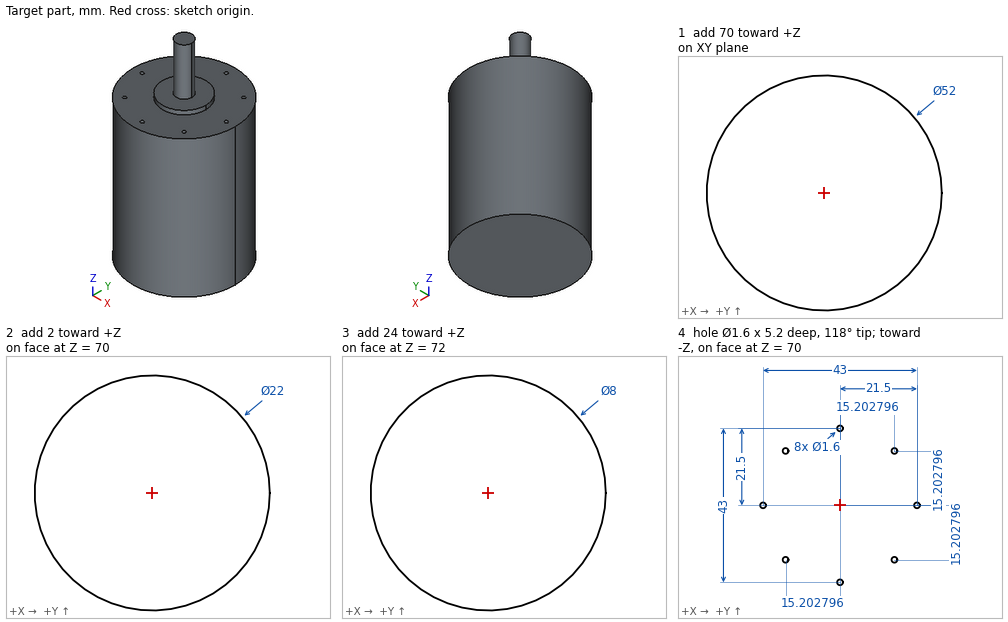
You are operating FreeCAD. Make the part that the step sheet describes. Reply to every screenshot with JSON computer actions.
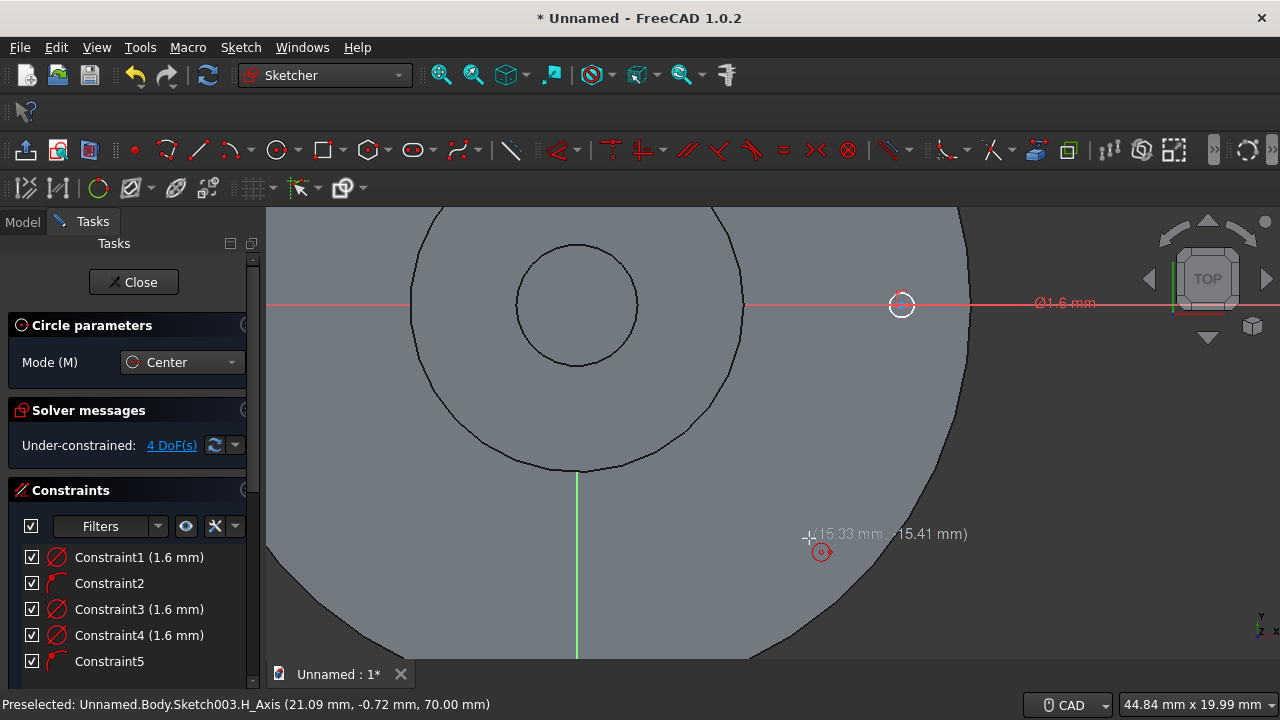
{"action": "left_click", "coordinate": [809, 537]}
{"action": "mouse_move", "coordinate": [812, 534]}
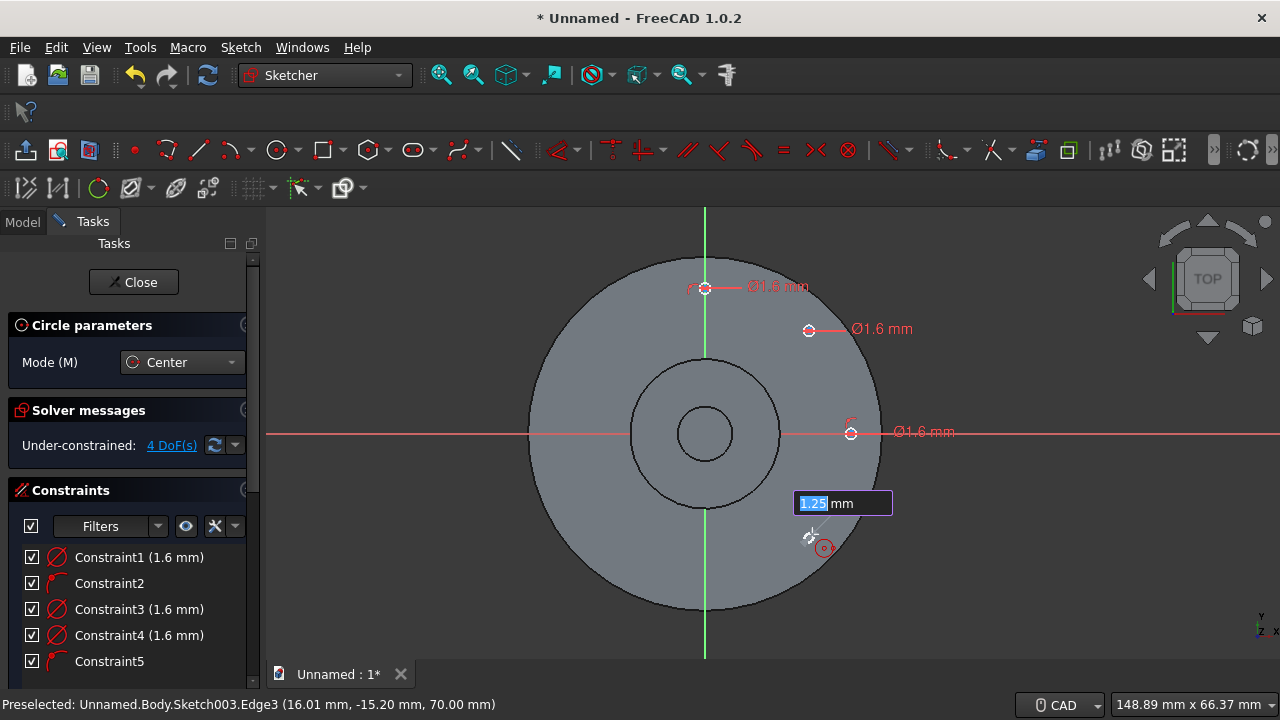
{"action": "type", "text": "1.6"}
{"action": "key", "text": "Return"}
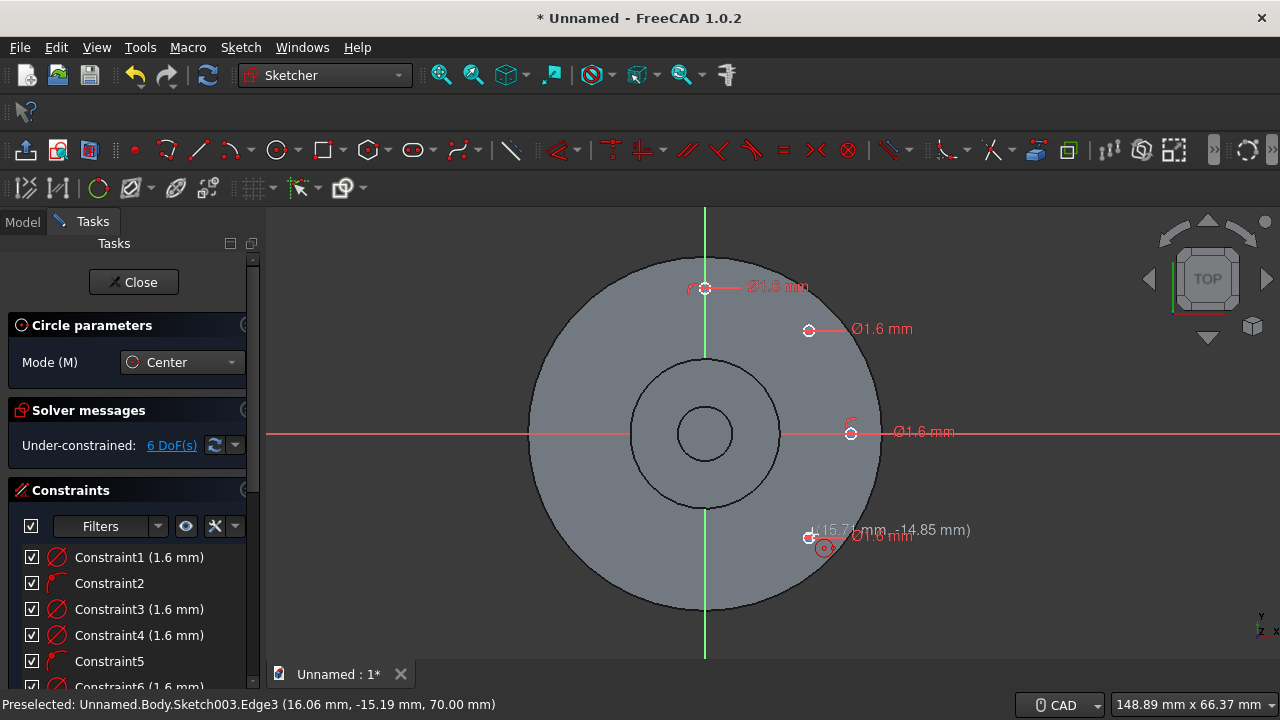
{"action": "scroll", "coordinate": [705, 580], "scroll_direction": "up", "scroll_amount": 8}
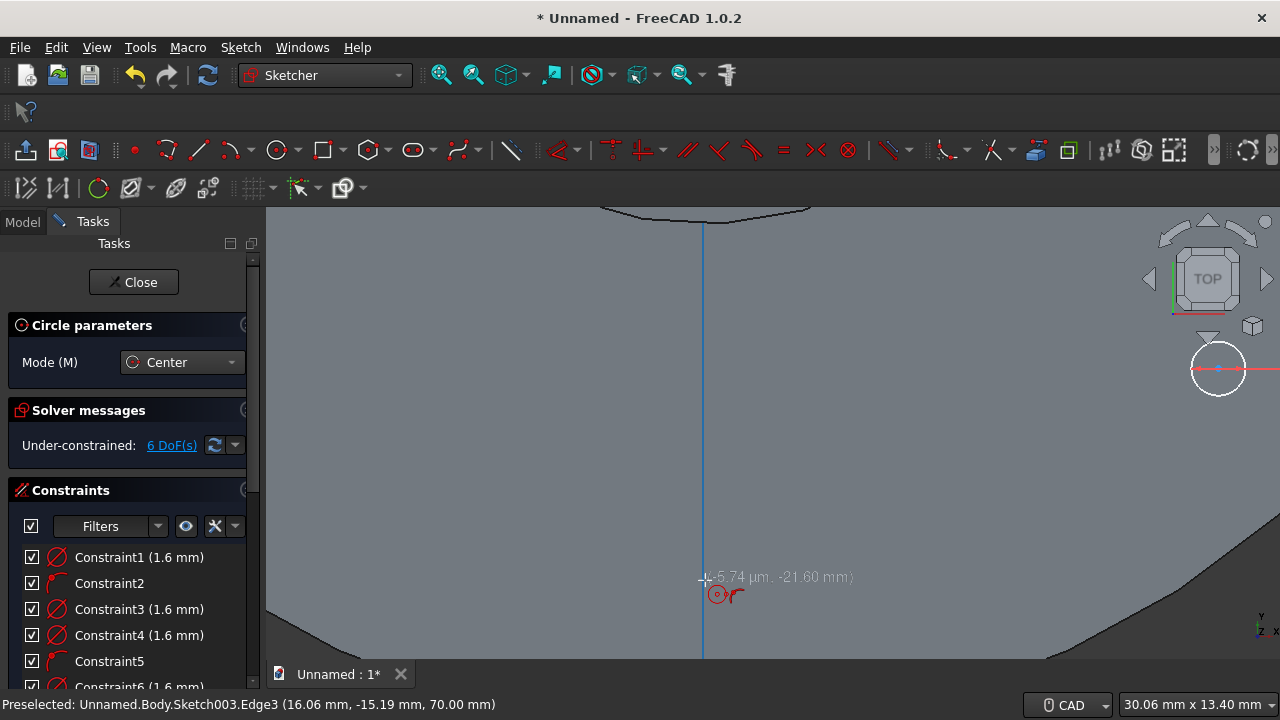
{"action": "scroll", "coordinate": [705, 580], "scroll_direction": "down", "scroll_amount": 8}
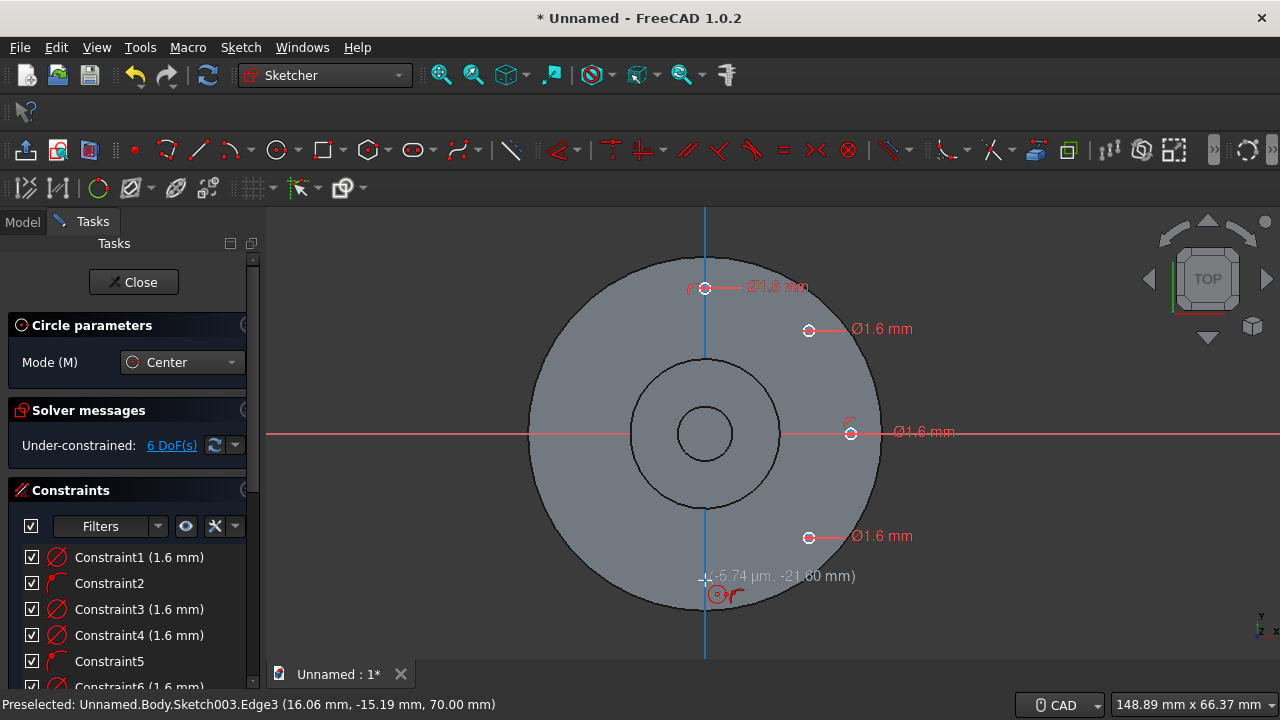
{"action": "left_click", "coordinate": [705, 580]}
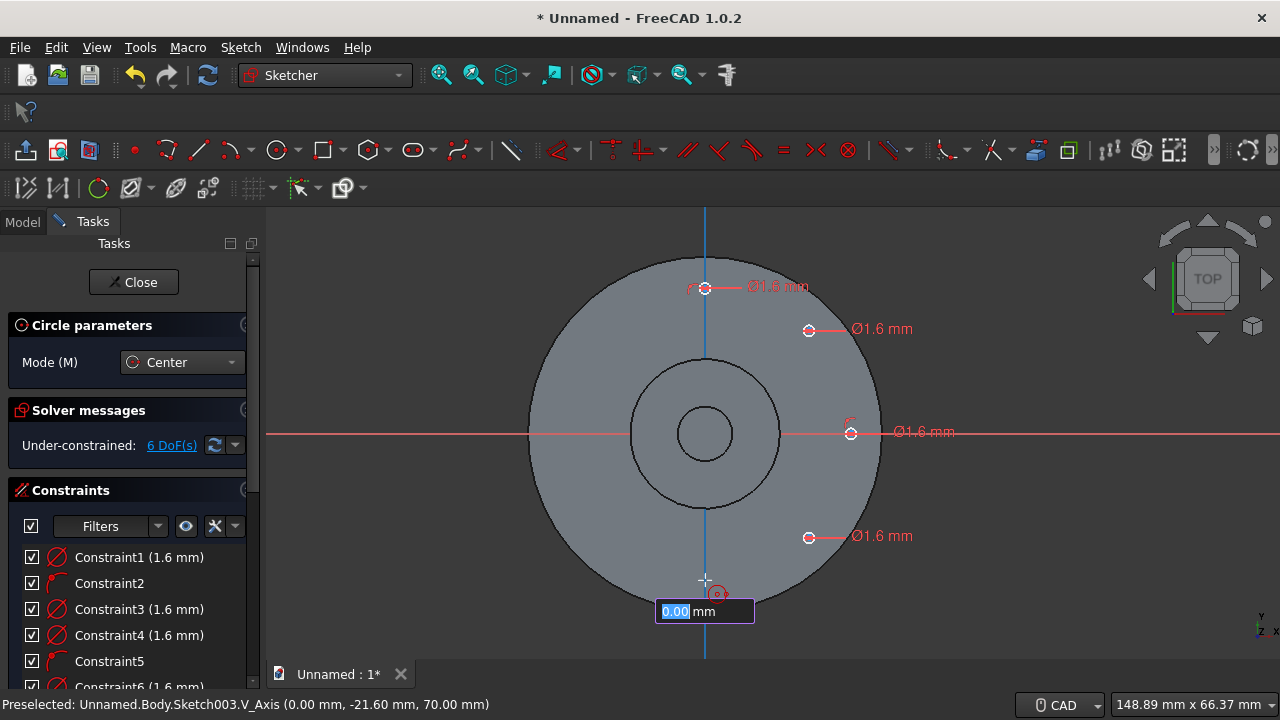
{"action": "scroll", "coordinate": [710, 578], "scroll_direction": "up", "scroll_amount": 6}
{"action": "mouse_move", "coordinate": [710, 577]}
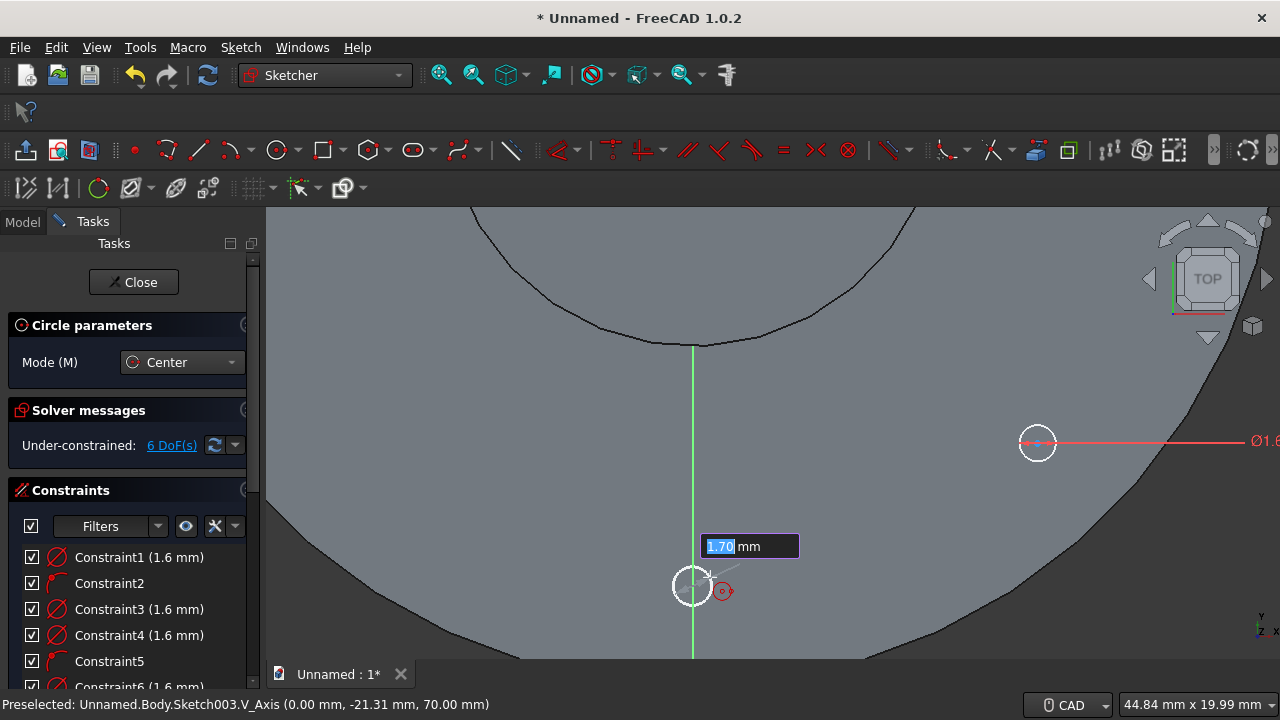
{"action": "type", "text": "1.6"}
{"action": "key", "text": "Return"}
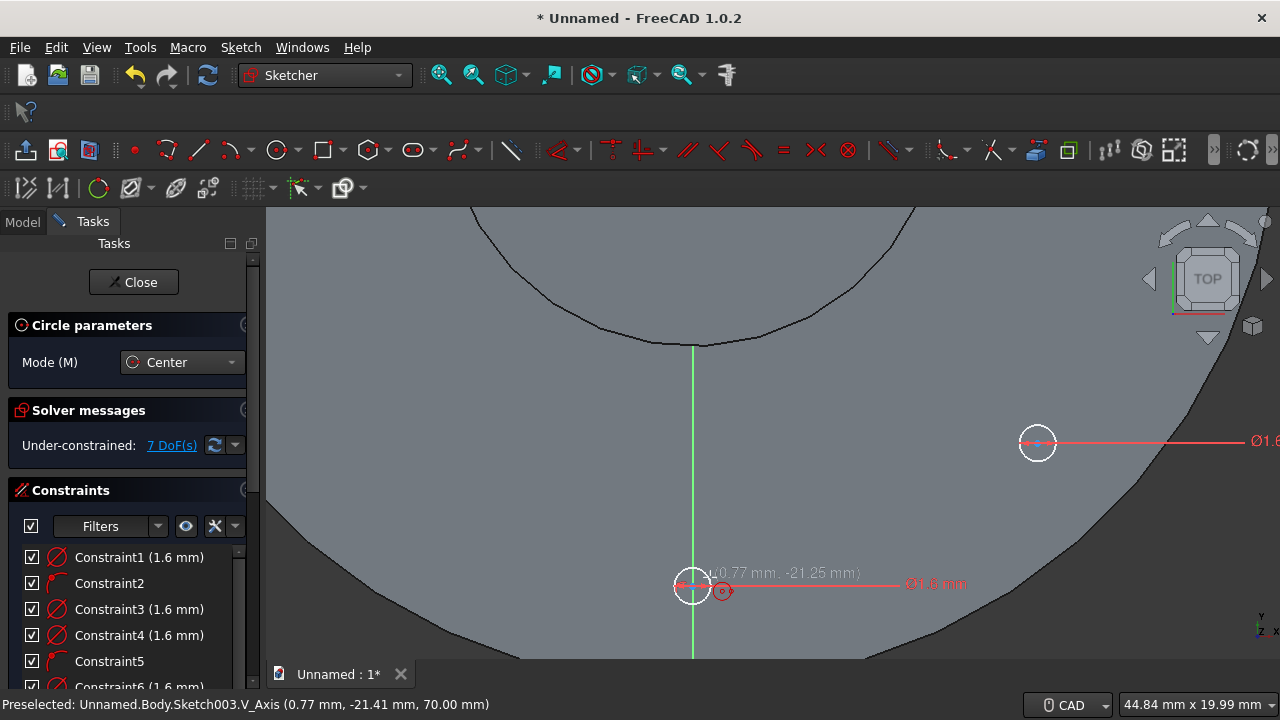
{"action": "scroll", "coordinate": [349, 441], "scroll_direction": "up", "scroll_amount": 2}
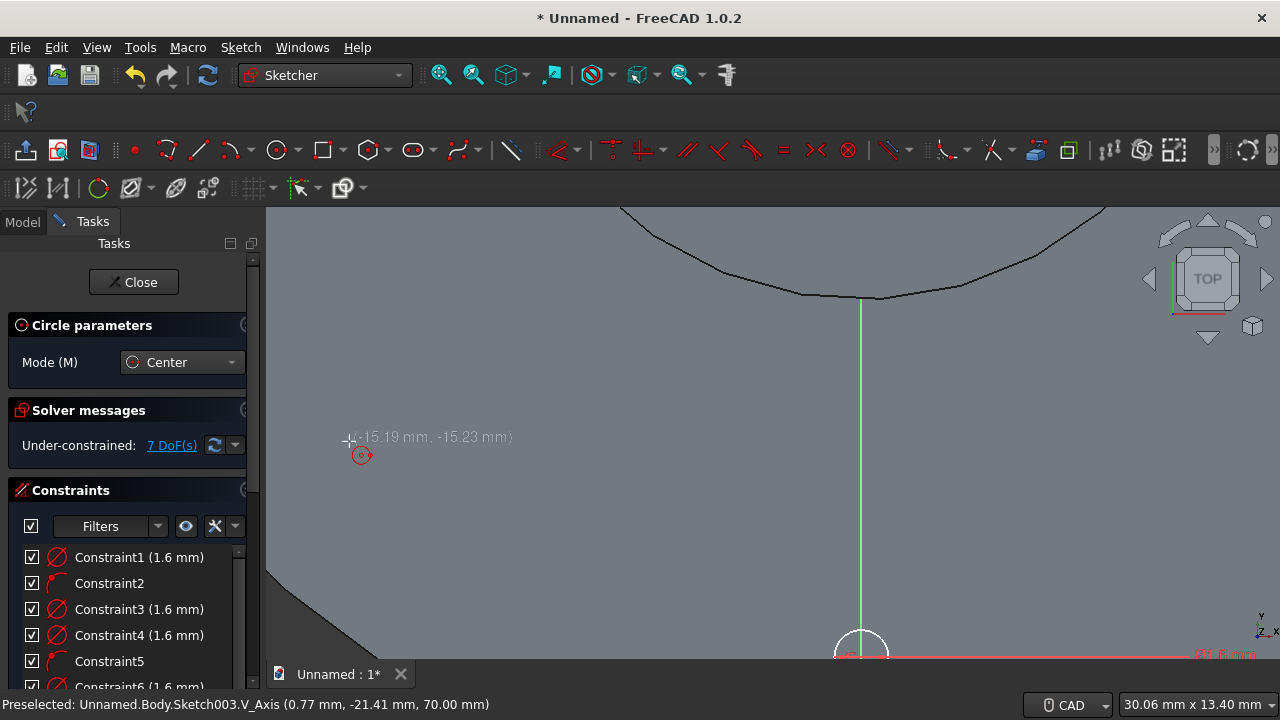
{"action": "scroll", "coordinate": [665, 561], "scroll_direction": "down", "scroll_amount": 8}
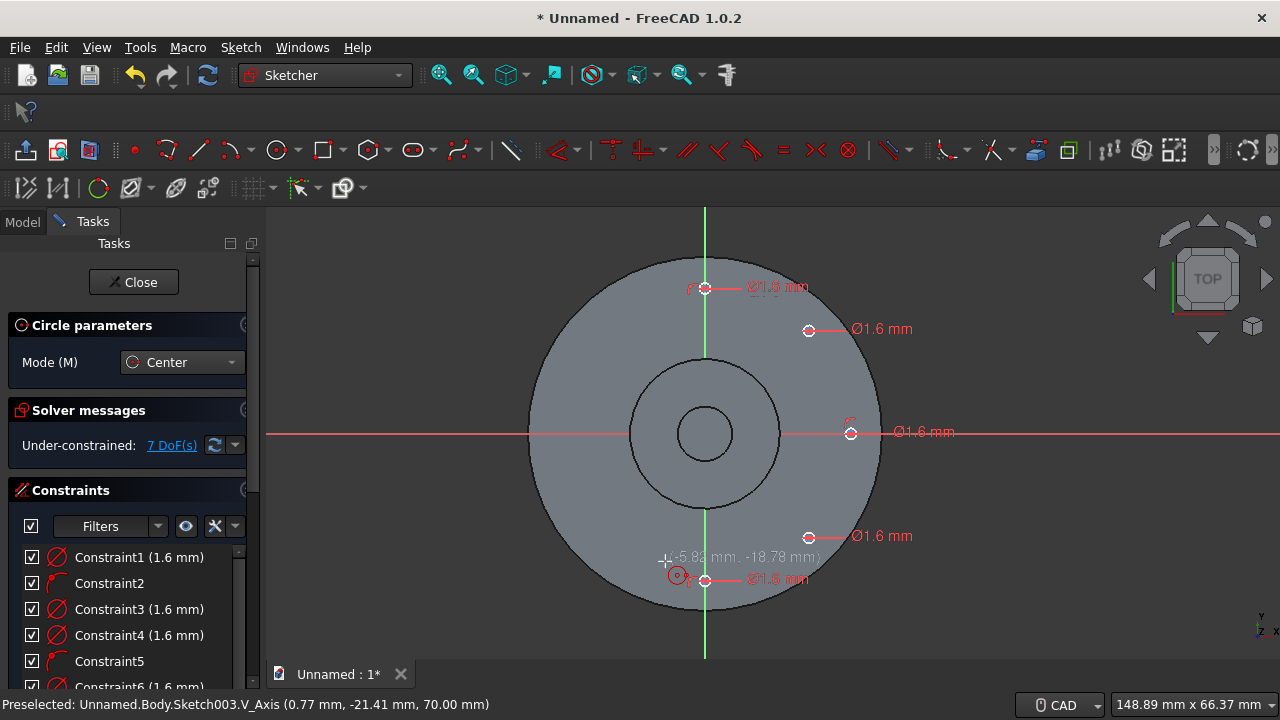
{"action": "left_click", "coordinate": [601, 537]}
{"action": "mouse_move", "coordinate": [605, 534]}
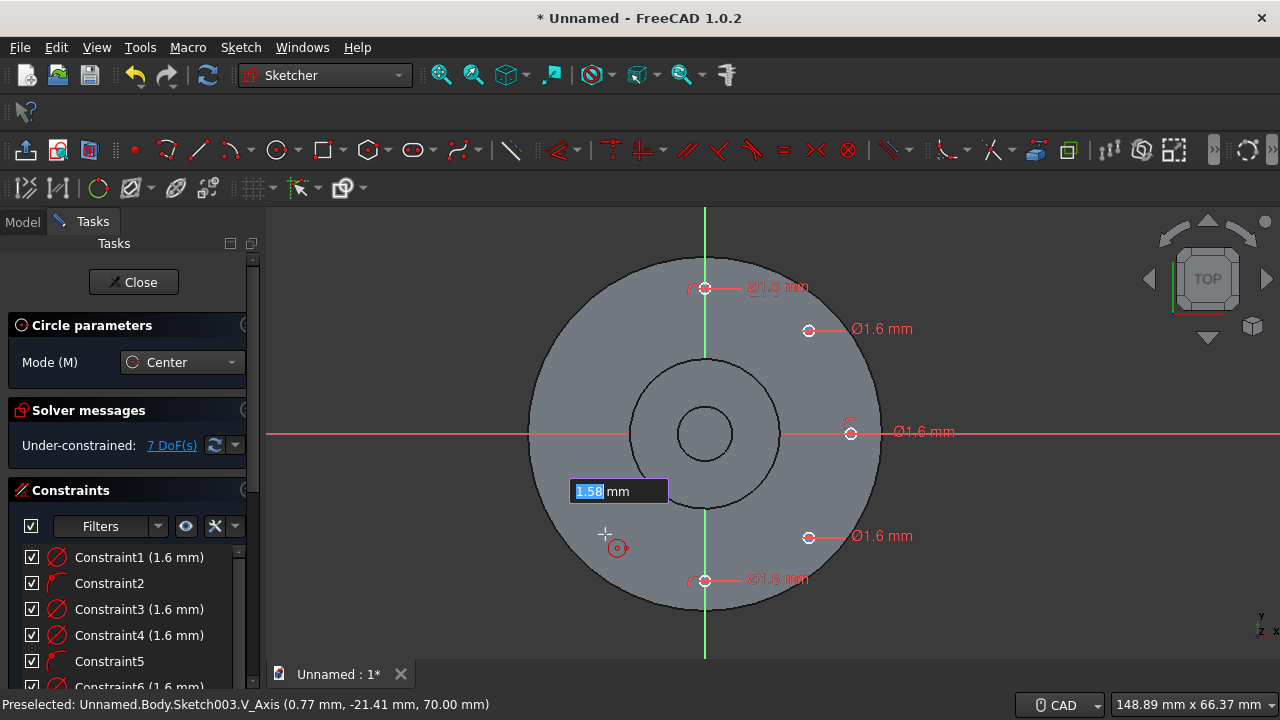
{"action": "type", "text": "1.6"}
{"action": "key", "text": "Return"}